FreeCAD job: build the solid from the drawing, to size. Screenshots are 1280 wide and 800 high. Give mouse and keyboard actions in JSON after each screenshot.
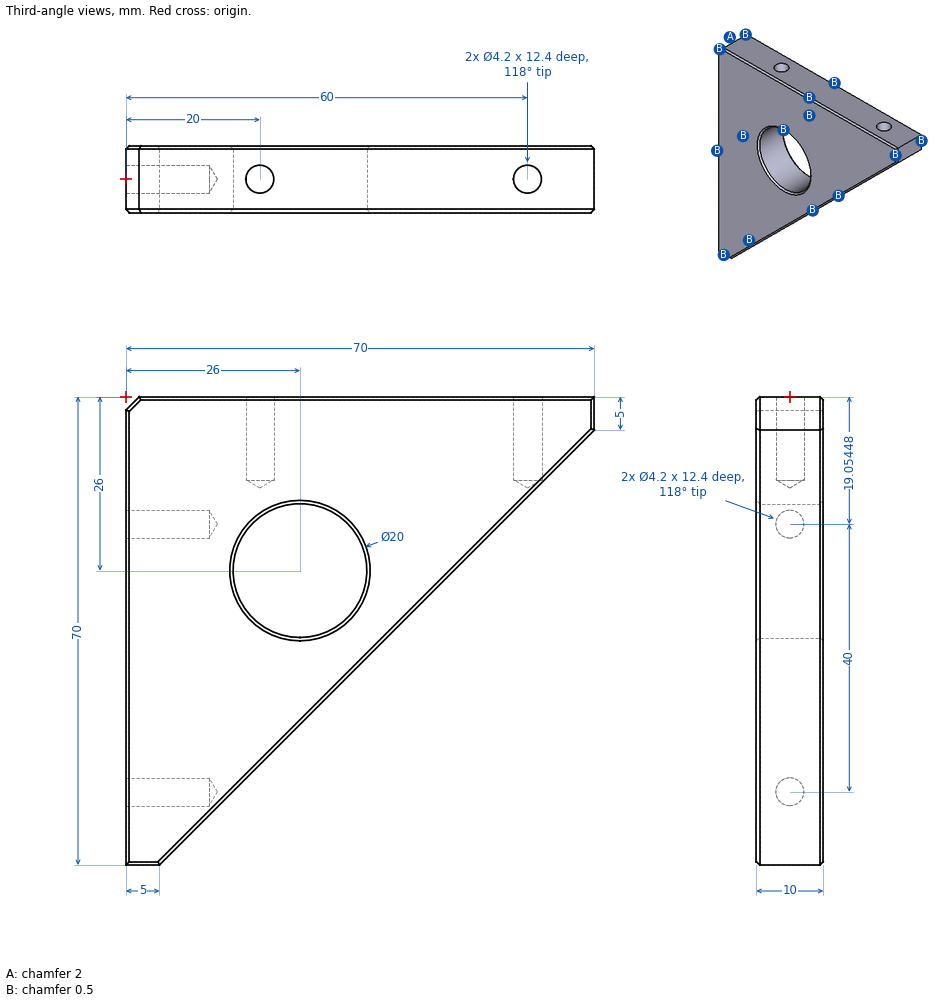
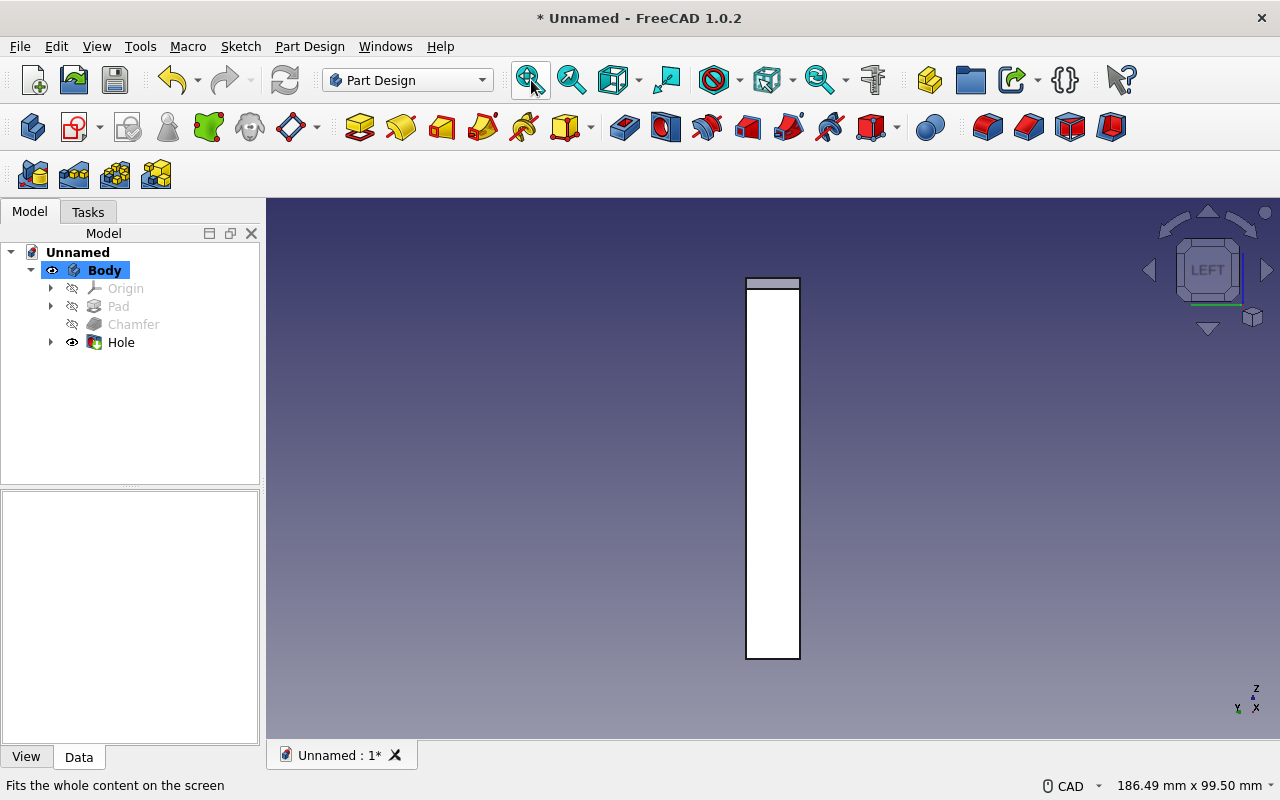
{"action": "left_click", "coordinate": [773, 367]}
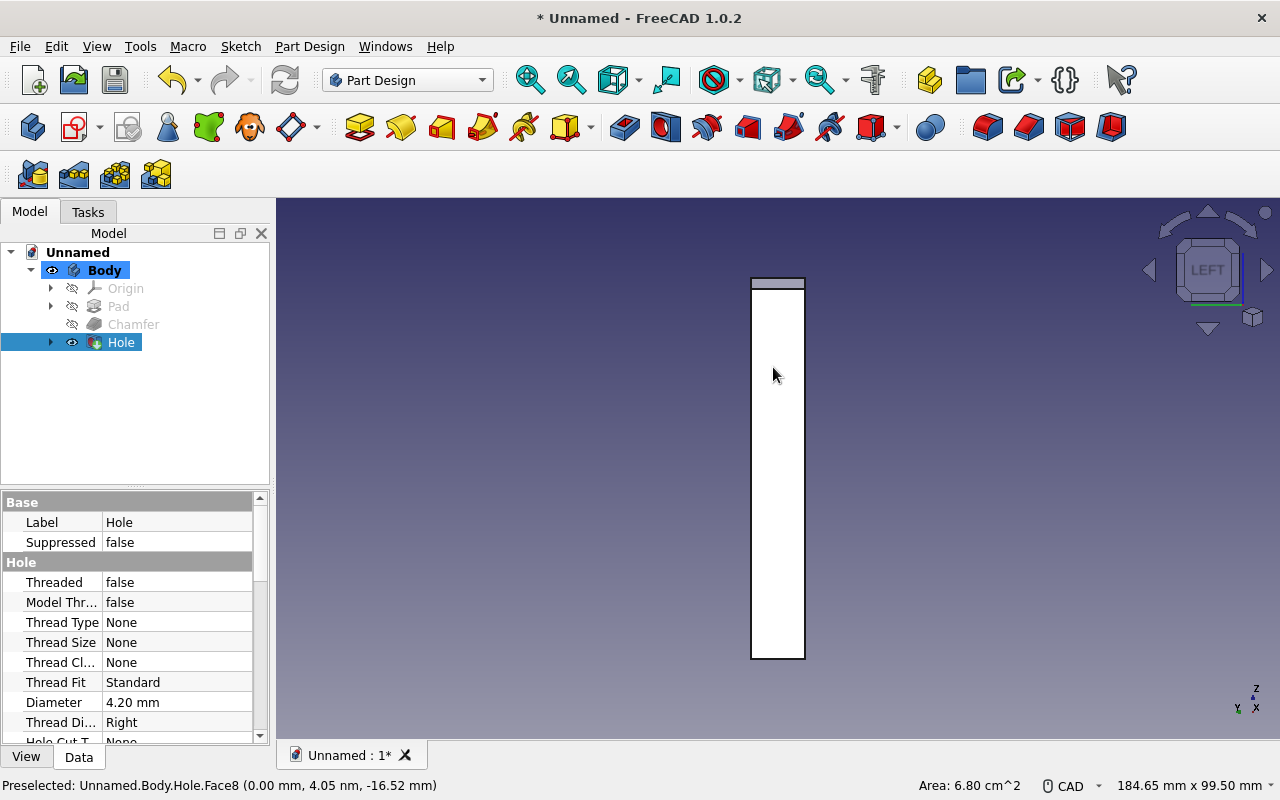
{"action": "left_click", "coordinate": [74, 128]}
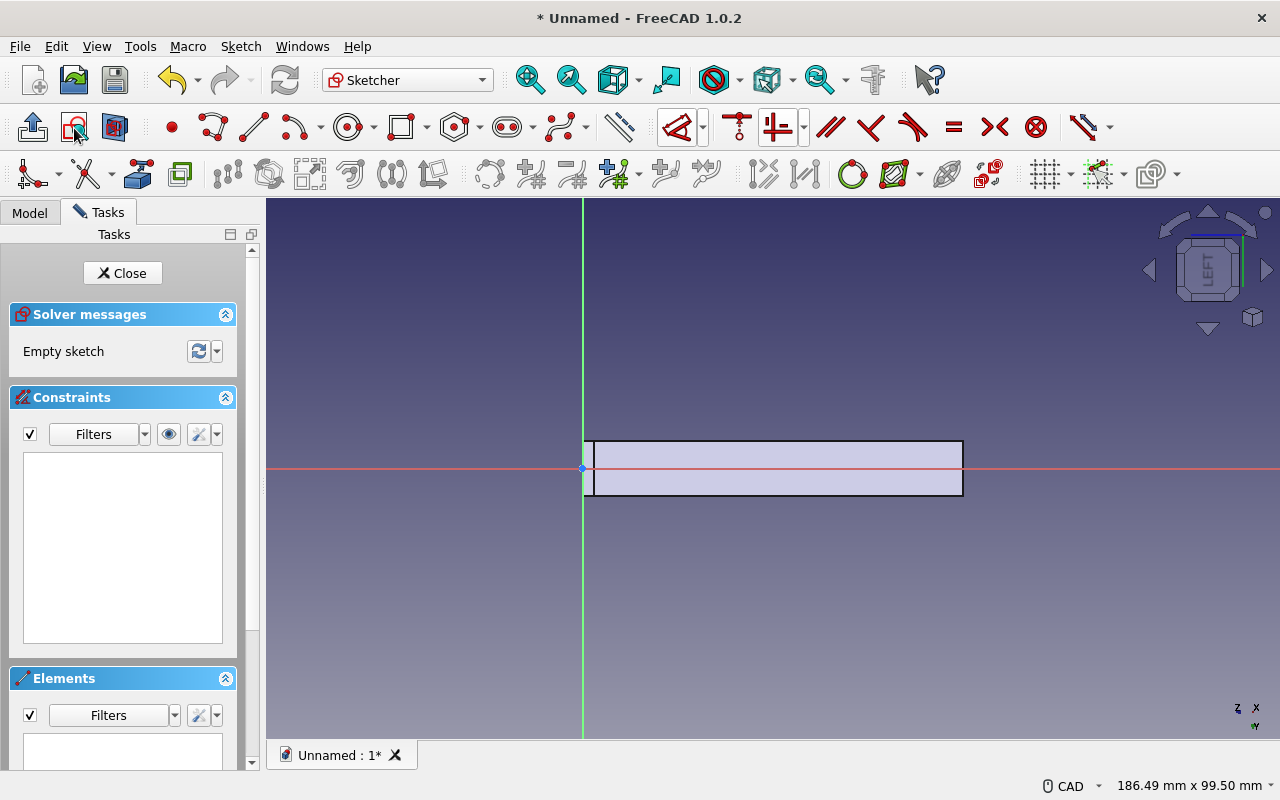
{"action": "scroll", "coordinate": [803, 468], "scroll_direction": "up", "scroll_amount": 3}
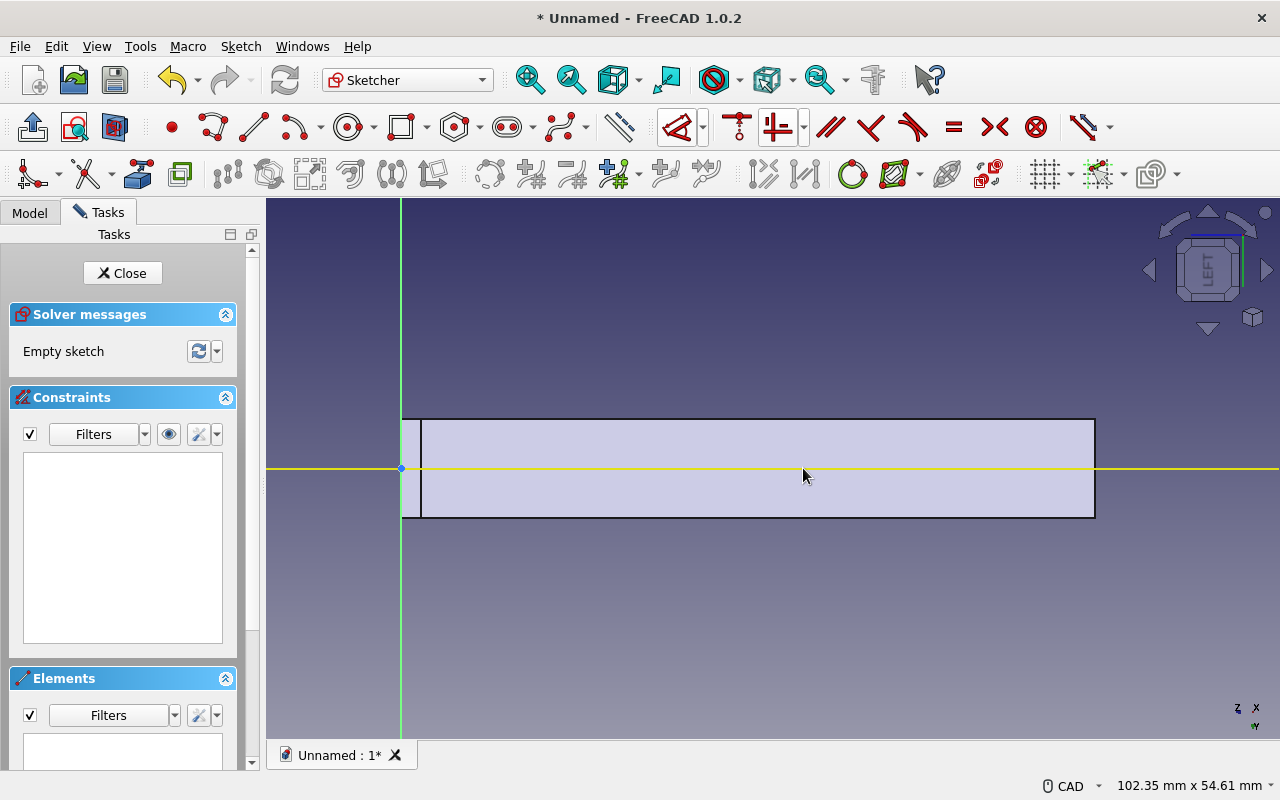
{"action": "left_click", "coordinate": [348, 128]}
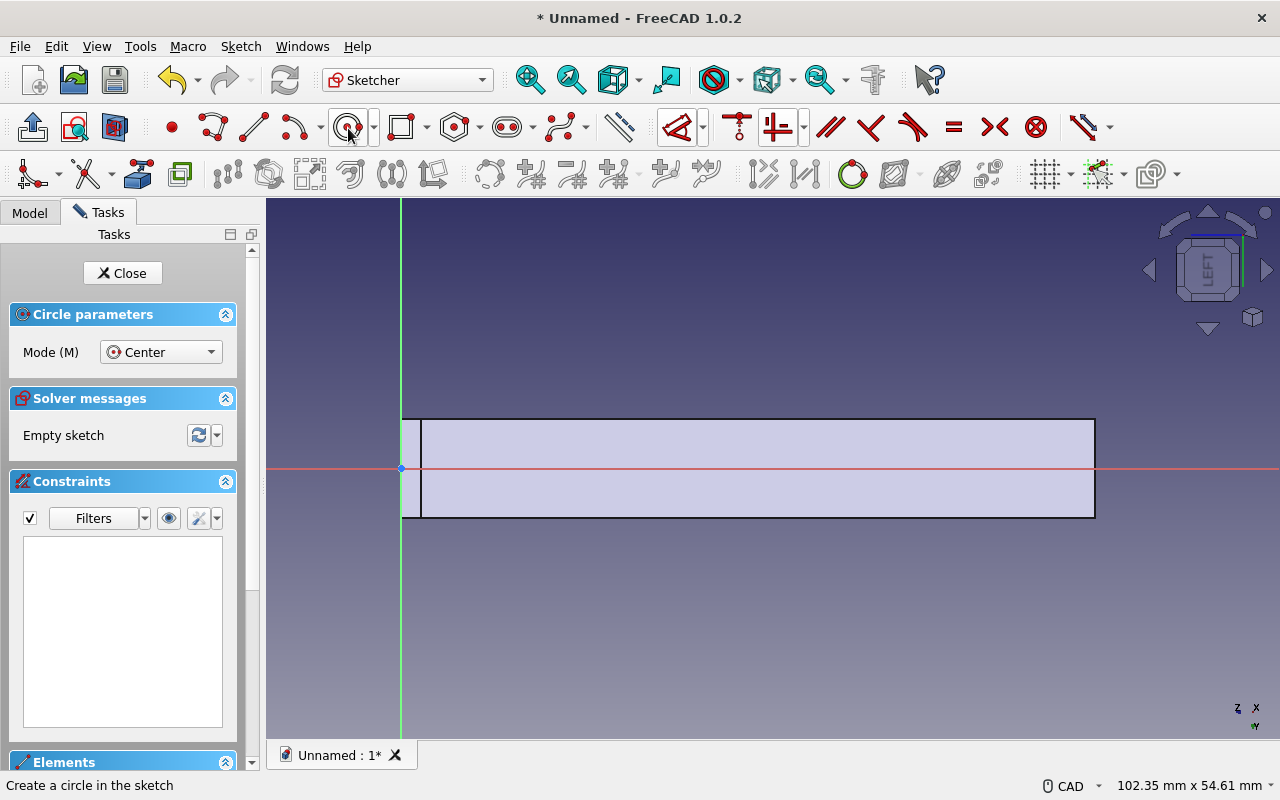
{"action": "left_click", "coordinate": [590, 468]}
{"action": "mouse_move", "coordinate": [605, 454]}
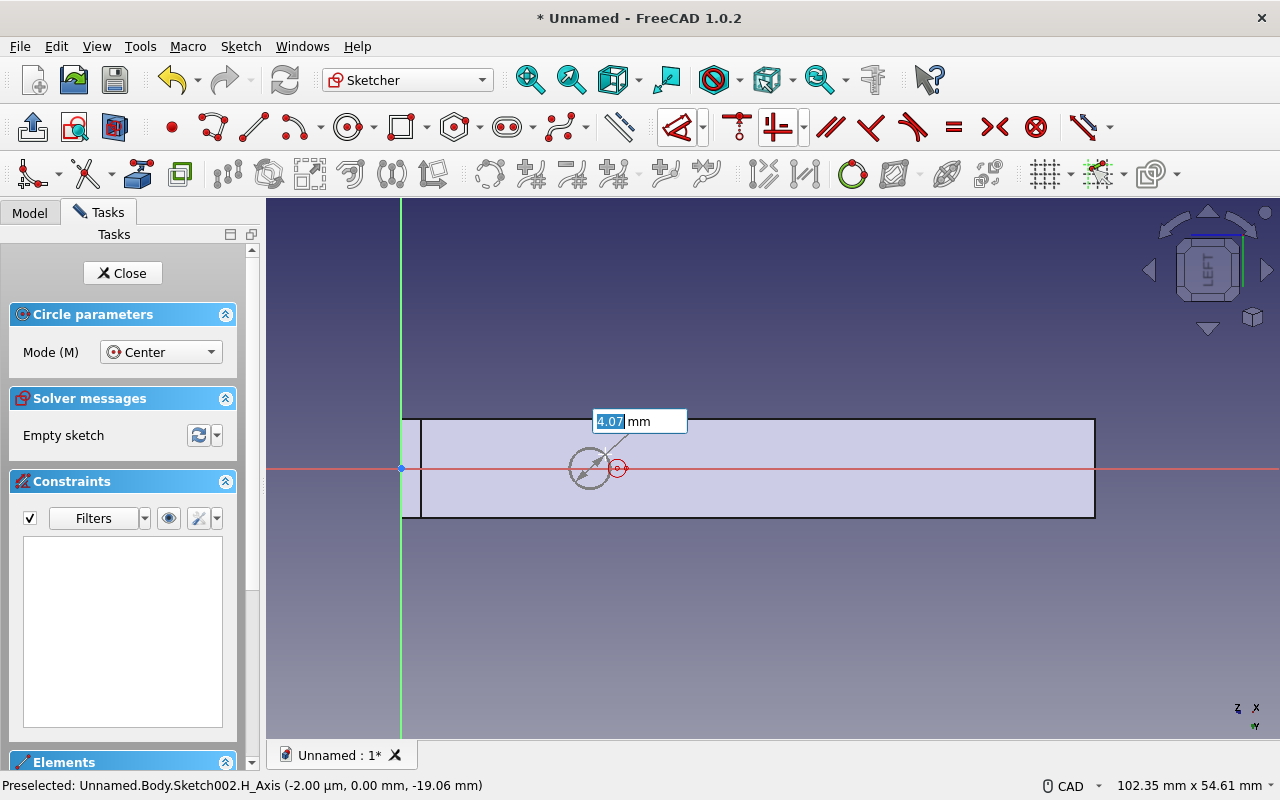
{"action": "type", "text": "4.2"}
{"action": "key", "text": "Return"}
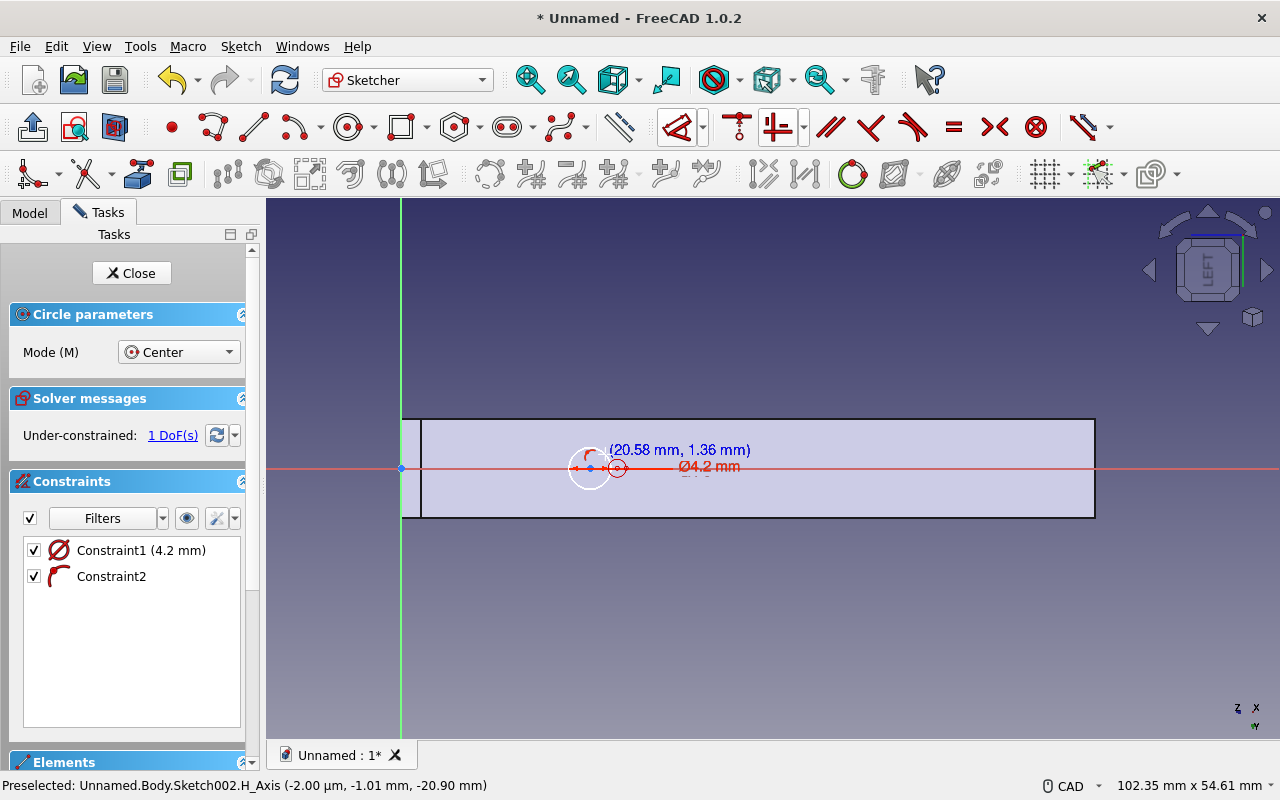
{"action": "left_click", "coordinate": [986, 468]}
{"action": "mouse_move", "coordinate": [1001, 454]}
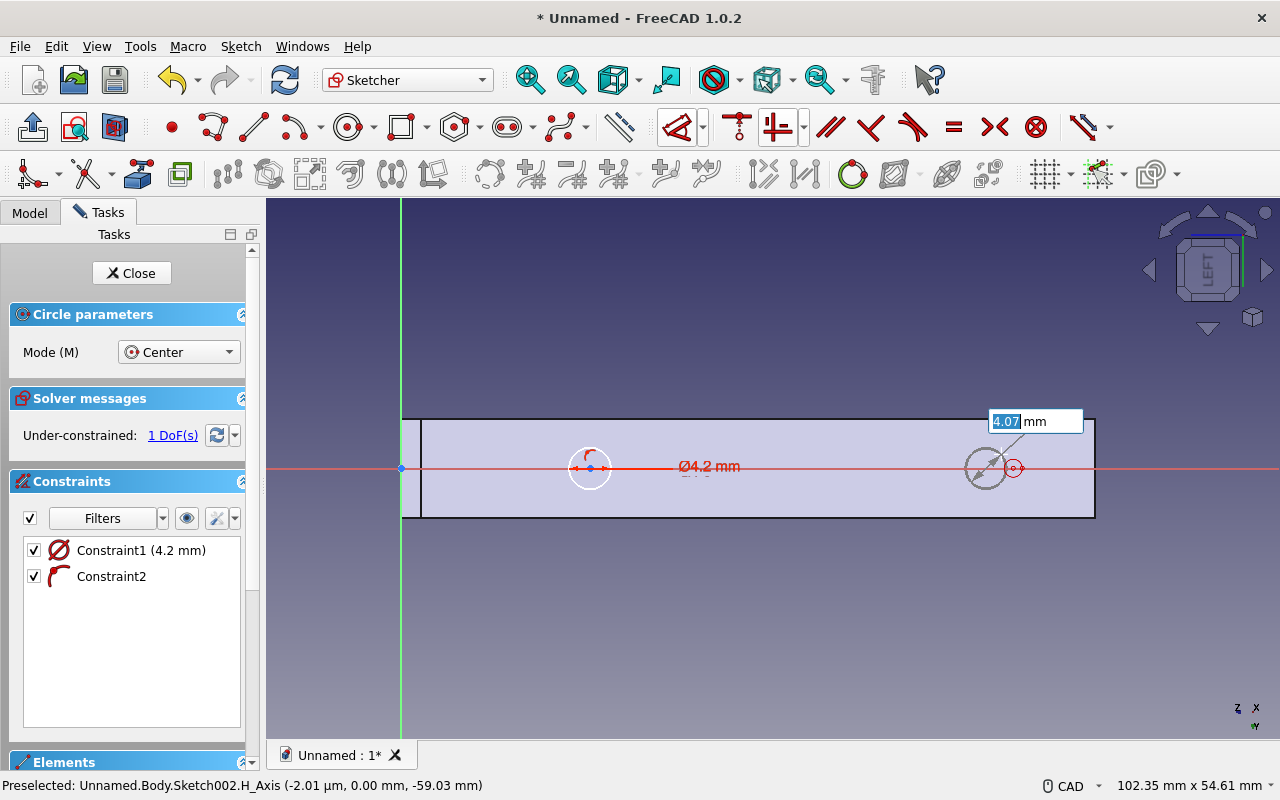
{"action": "type", "text": "4.2"}
{"action": "key", "text": "Return"}
{"action": "key", "text": "Escape"}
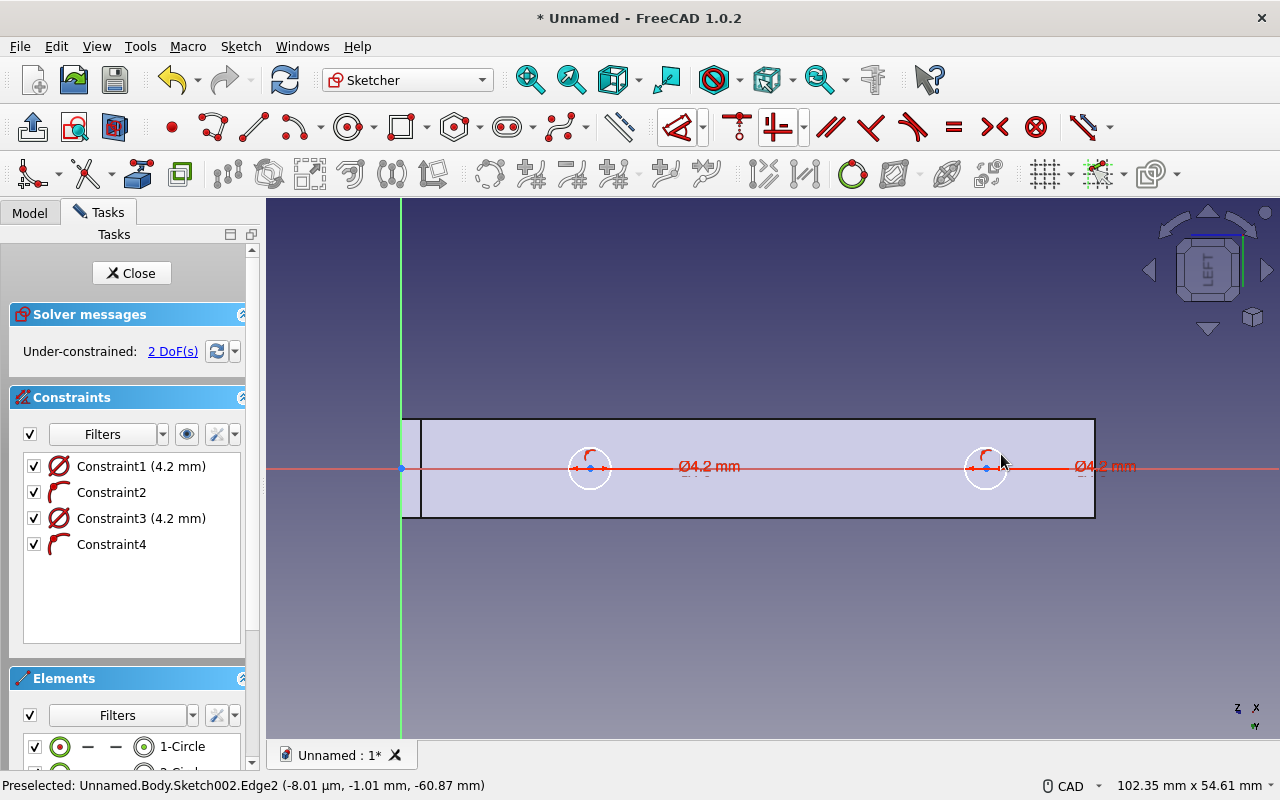
{"action": "left_click", "coordinate": [590, 468]}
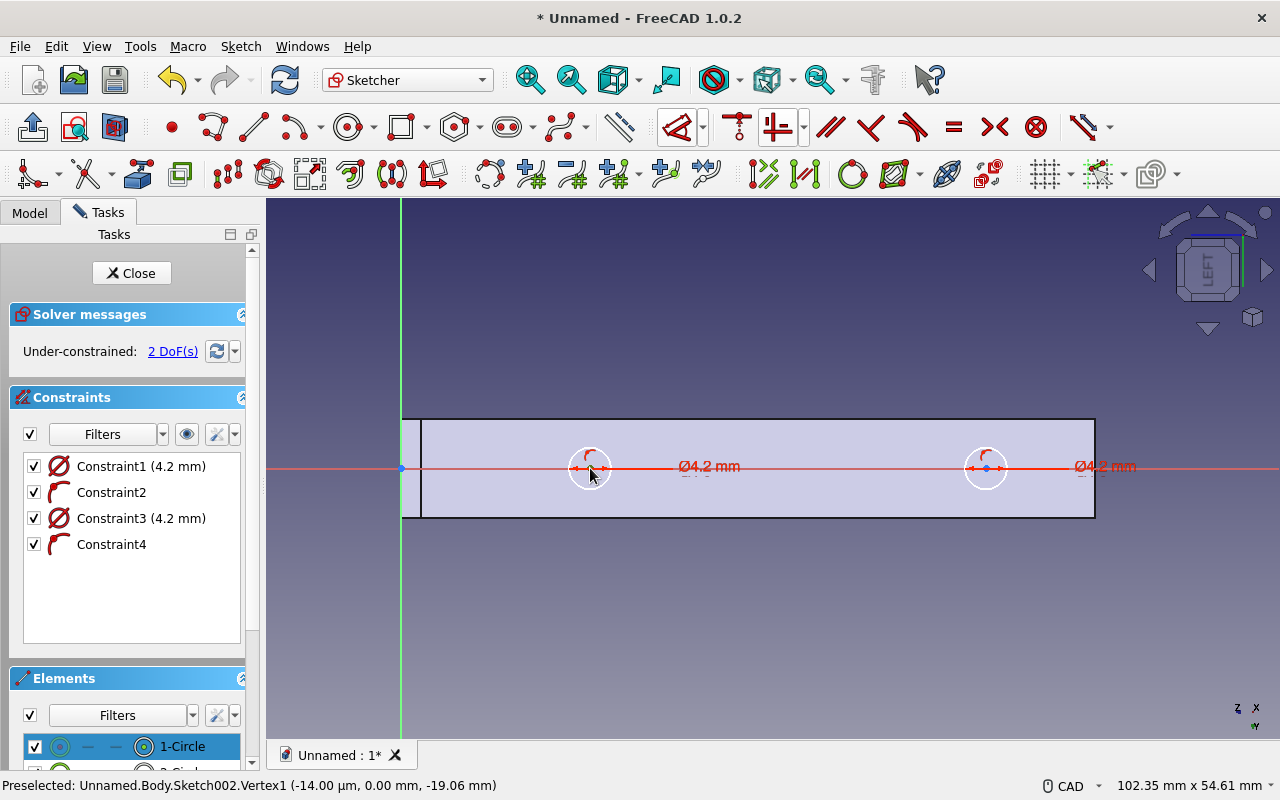
{"action": "left_click", "coordinate": [986, 468]}